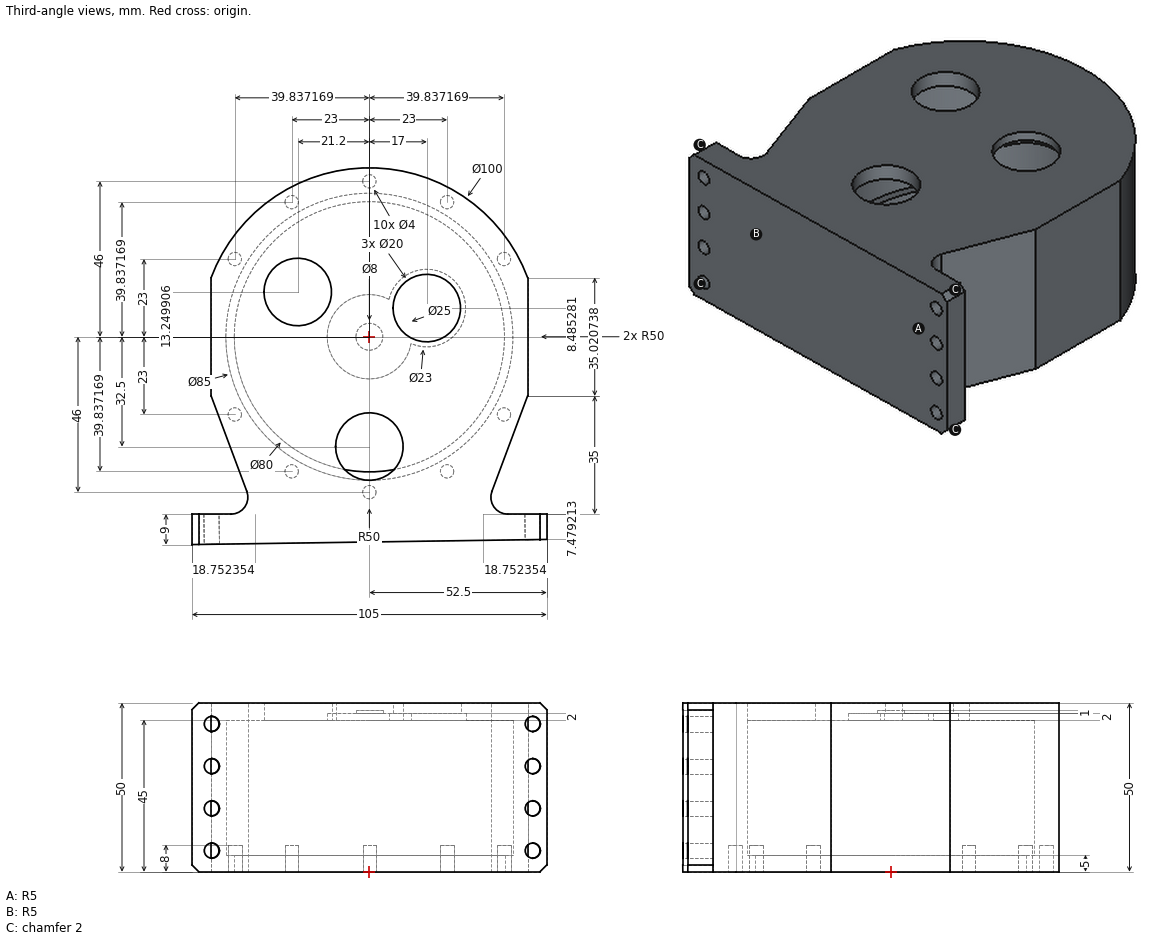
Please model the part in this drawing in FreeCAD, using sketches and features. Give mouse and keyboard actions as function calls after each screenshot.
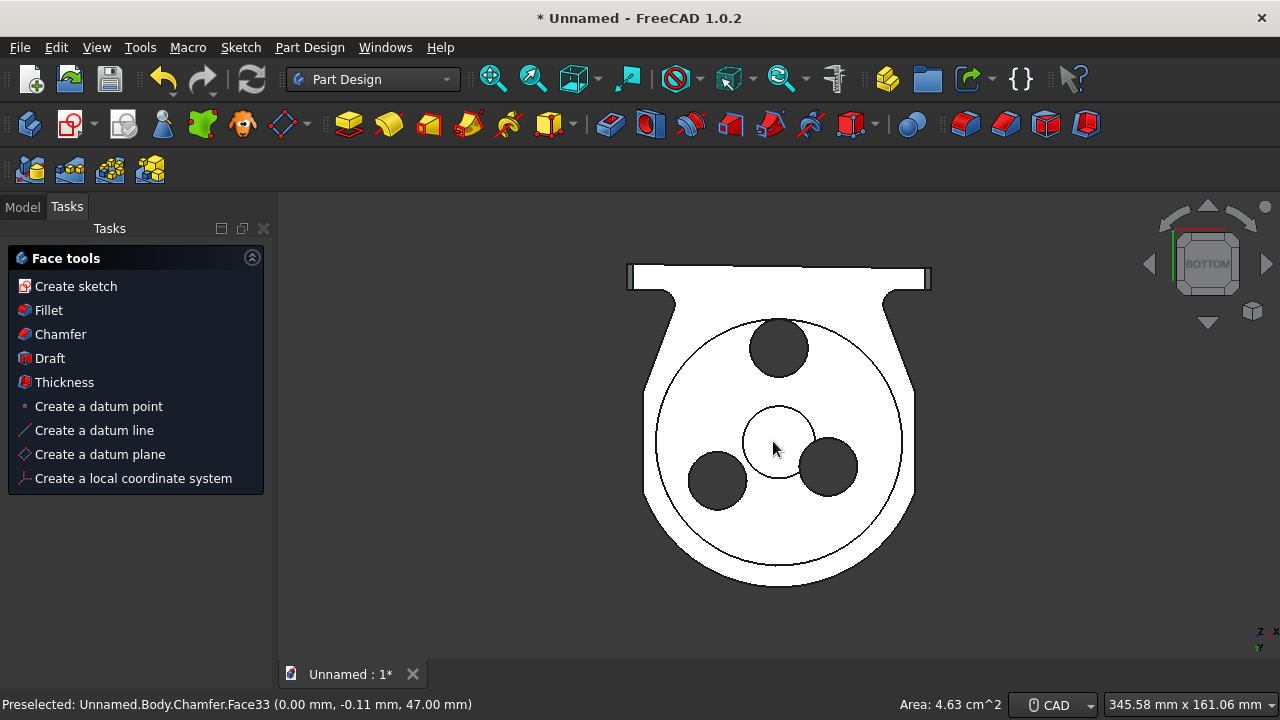
click(70, 124)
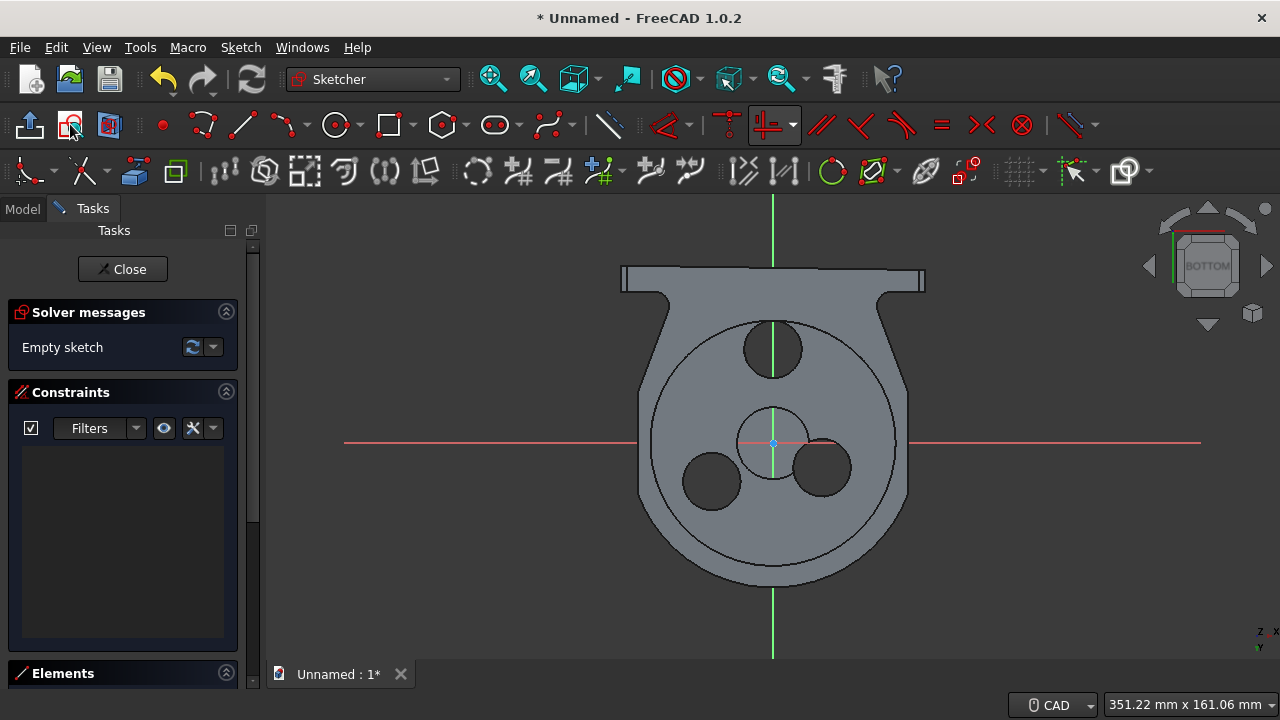
scroll(778, 445, up, 13)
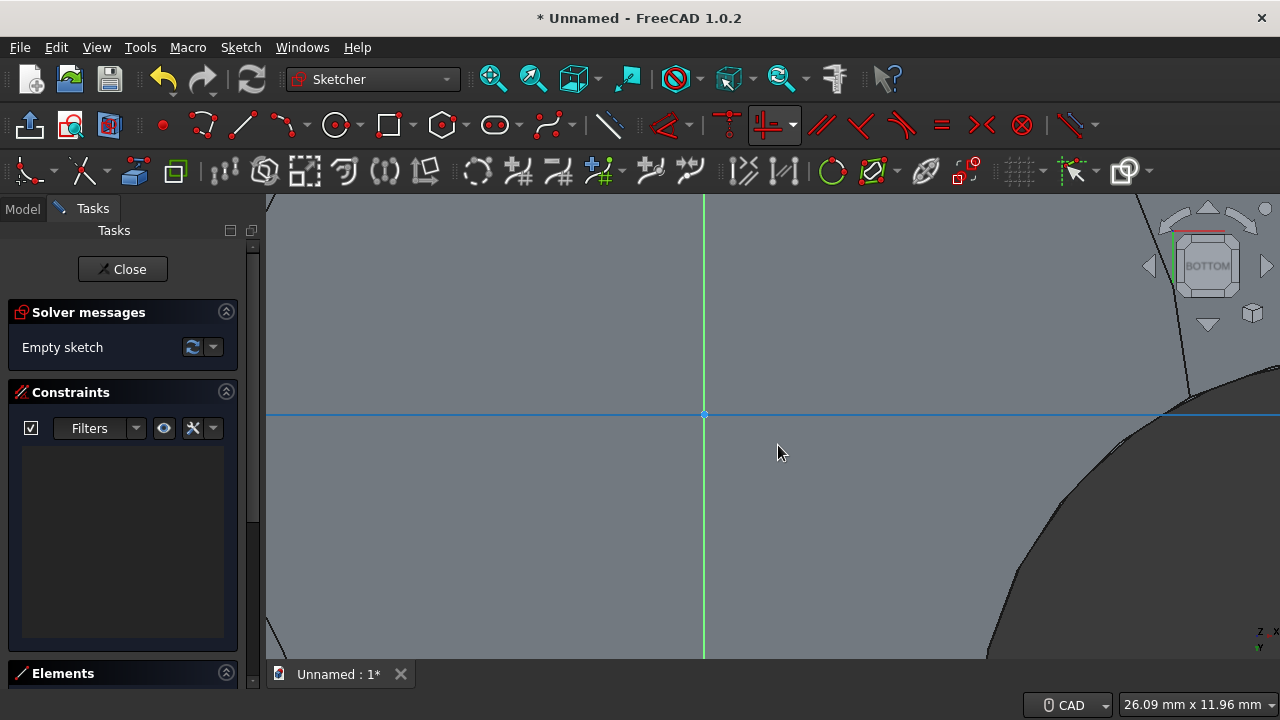
click(336, 126)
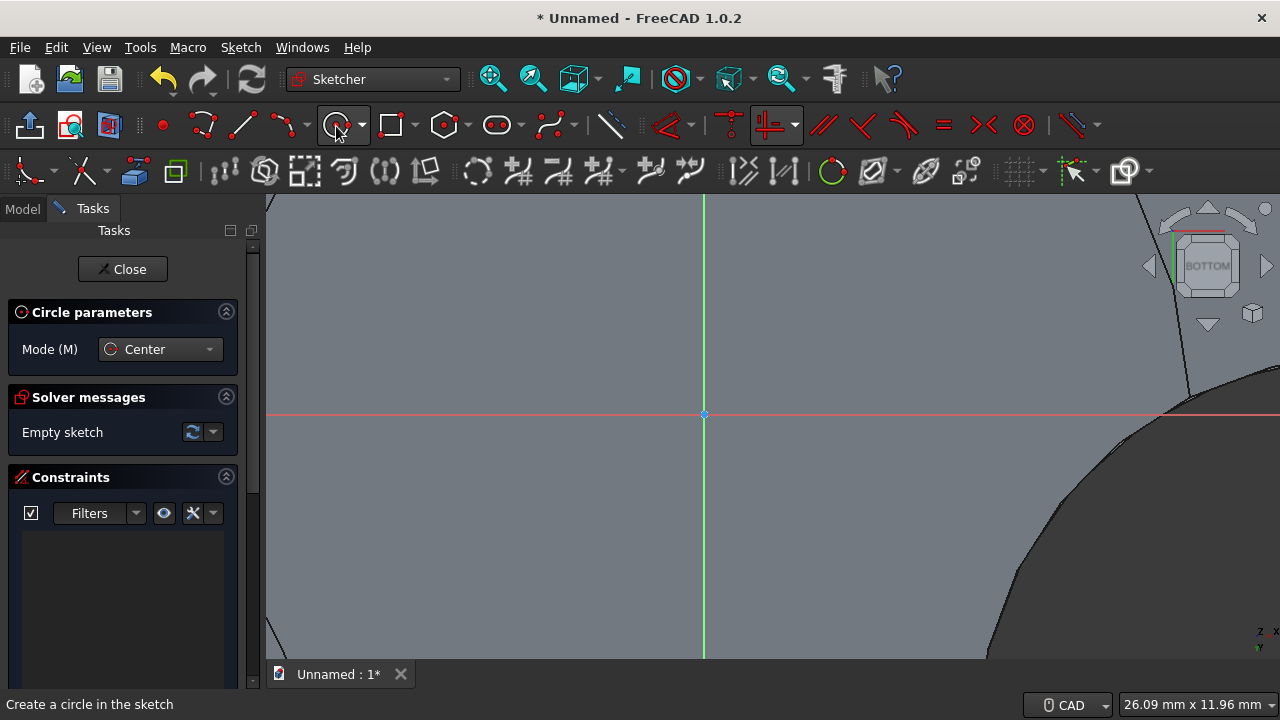
click(704, 415)
click(814, 305)
key(Escape)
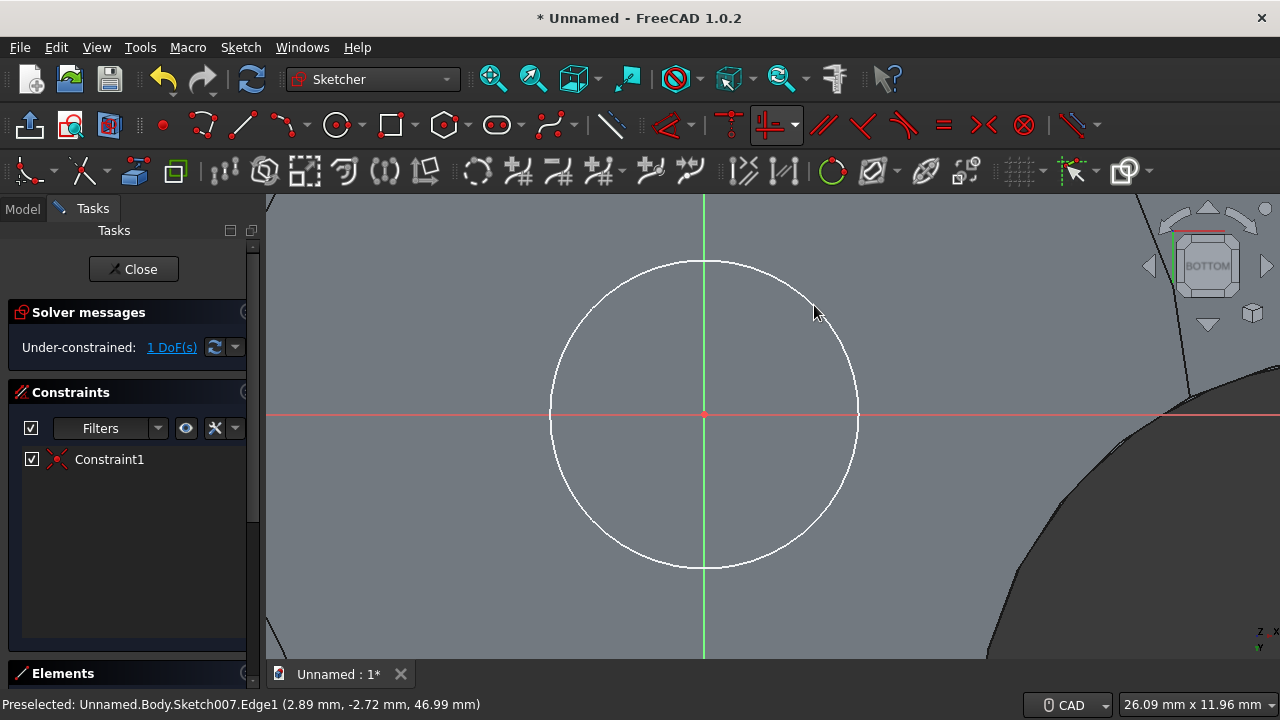
click(666, 126)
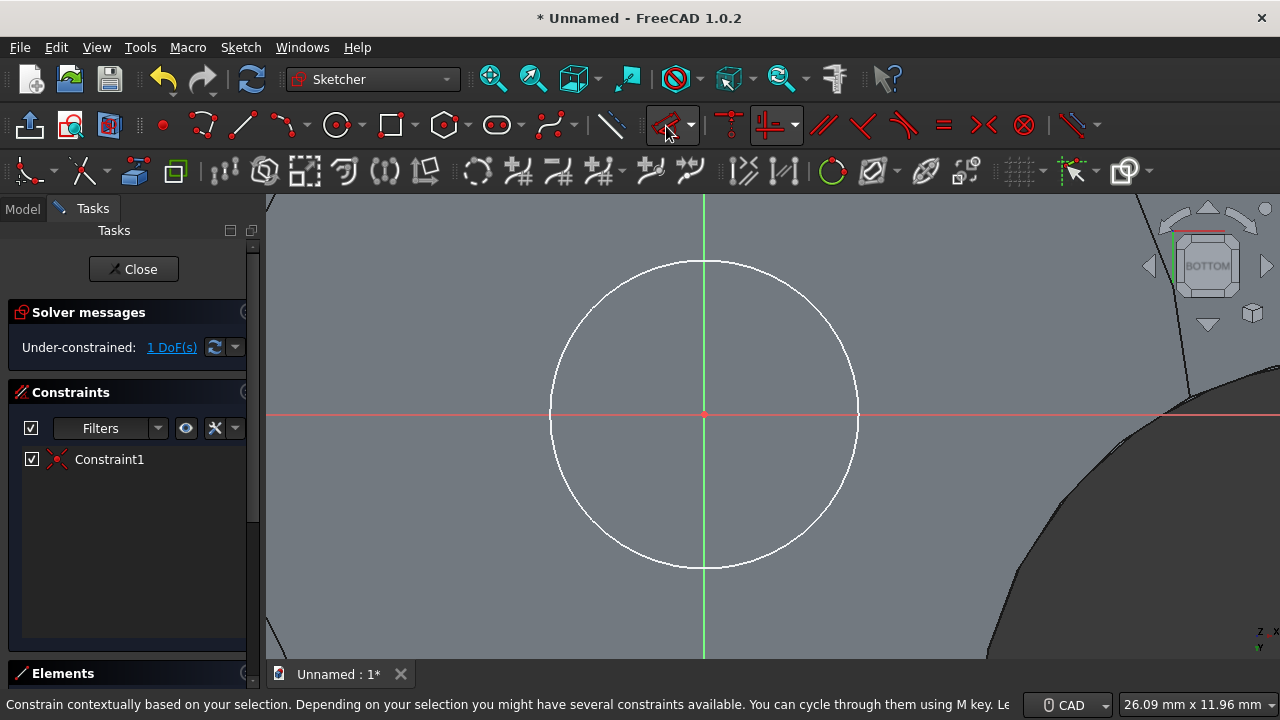
click(813, 305)
click(836, 282)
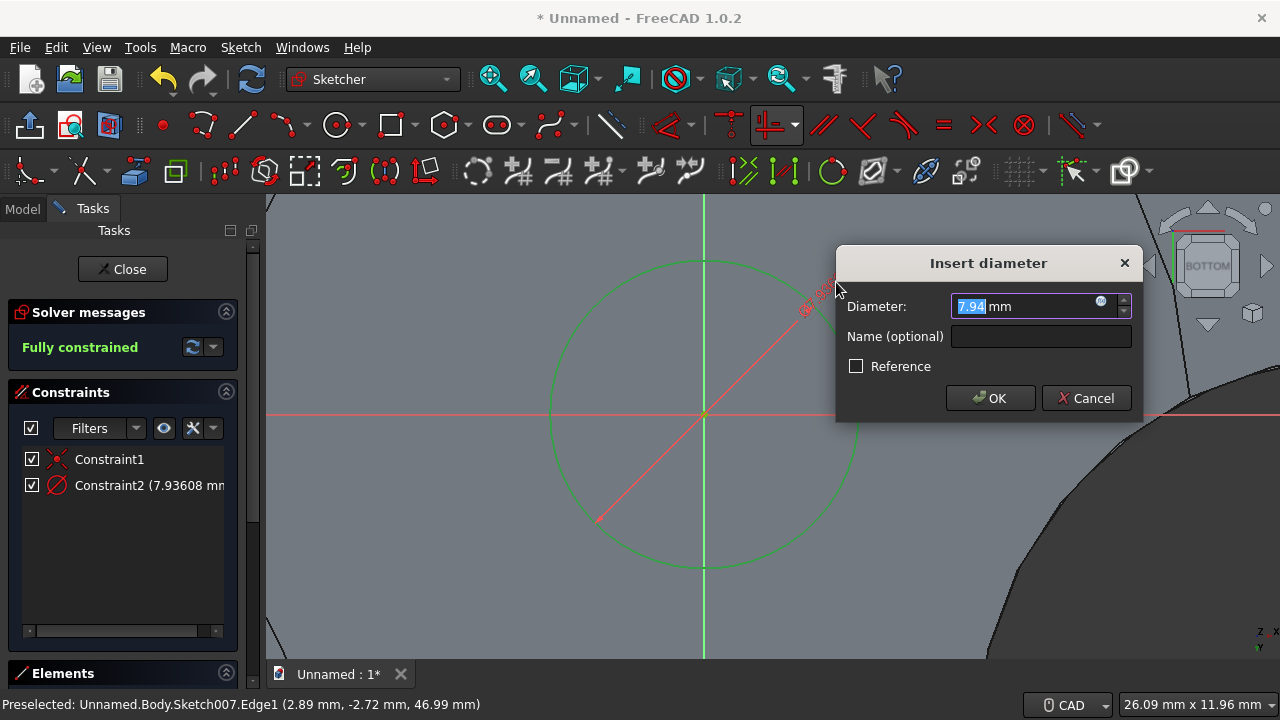
text(8)
key(Return)
key(Escape)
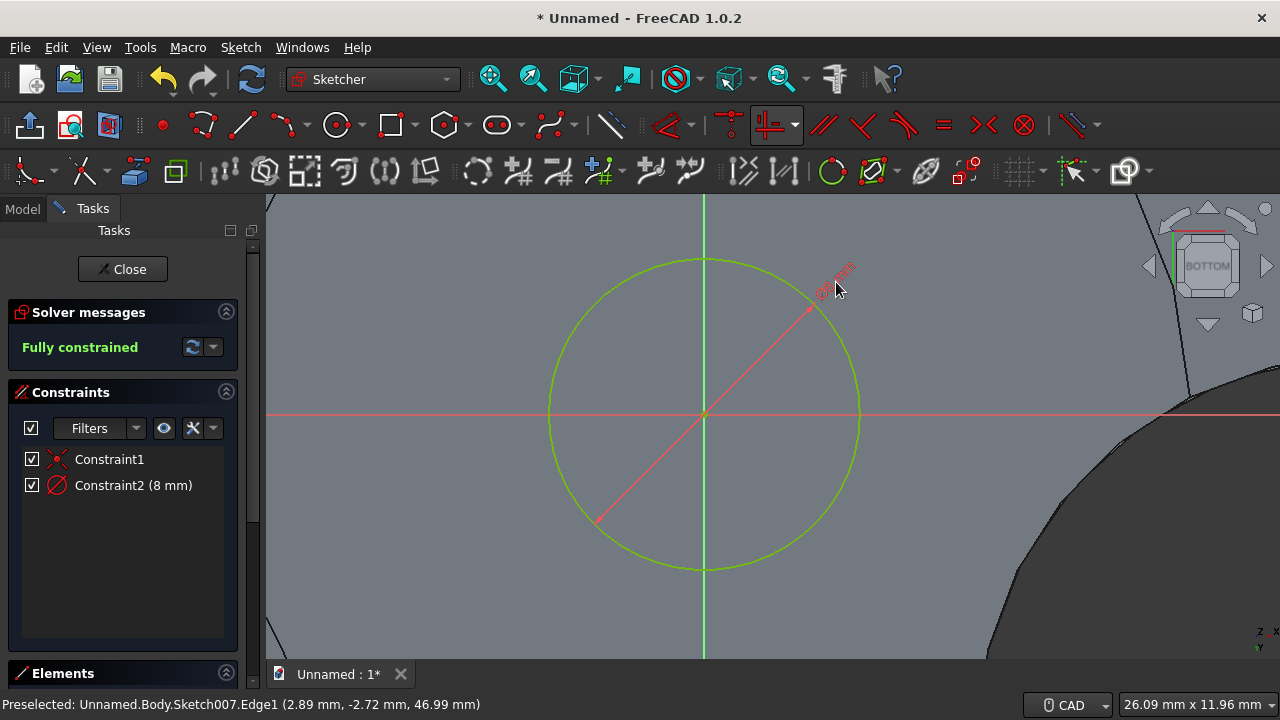
click(123, 269)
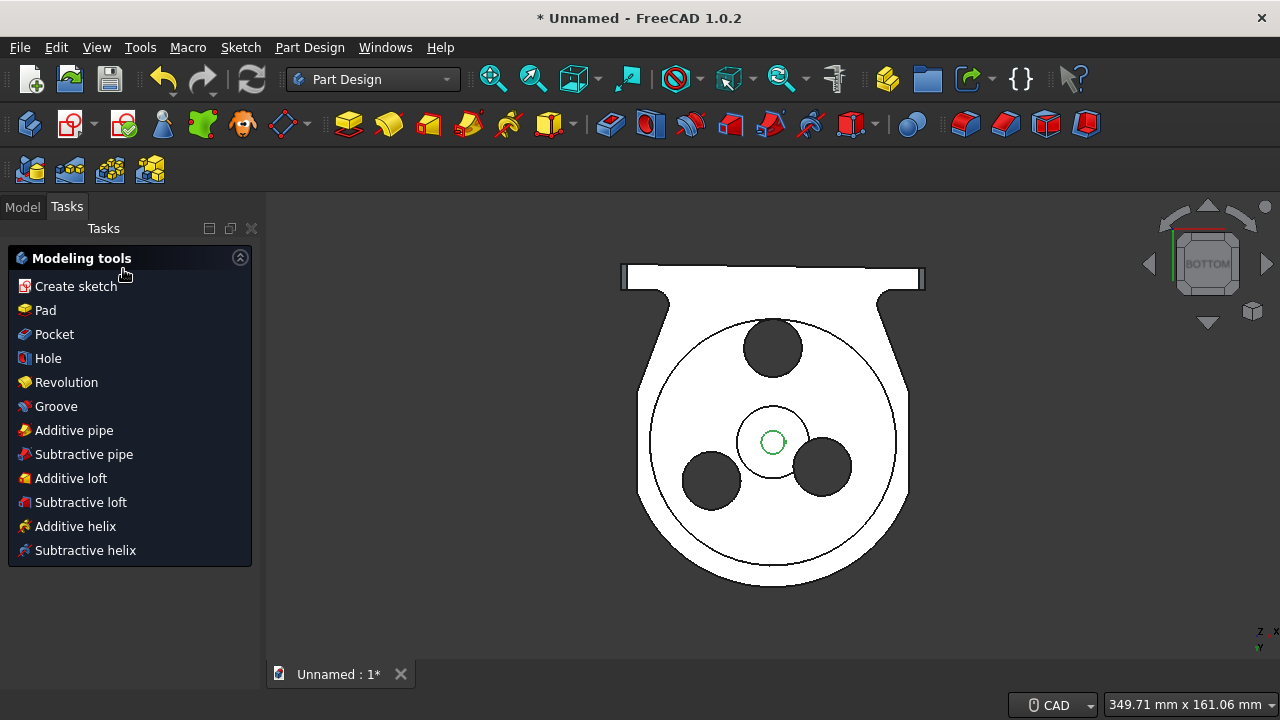
click(612, 124)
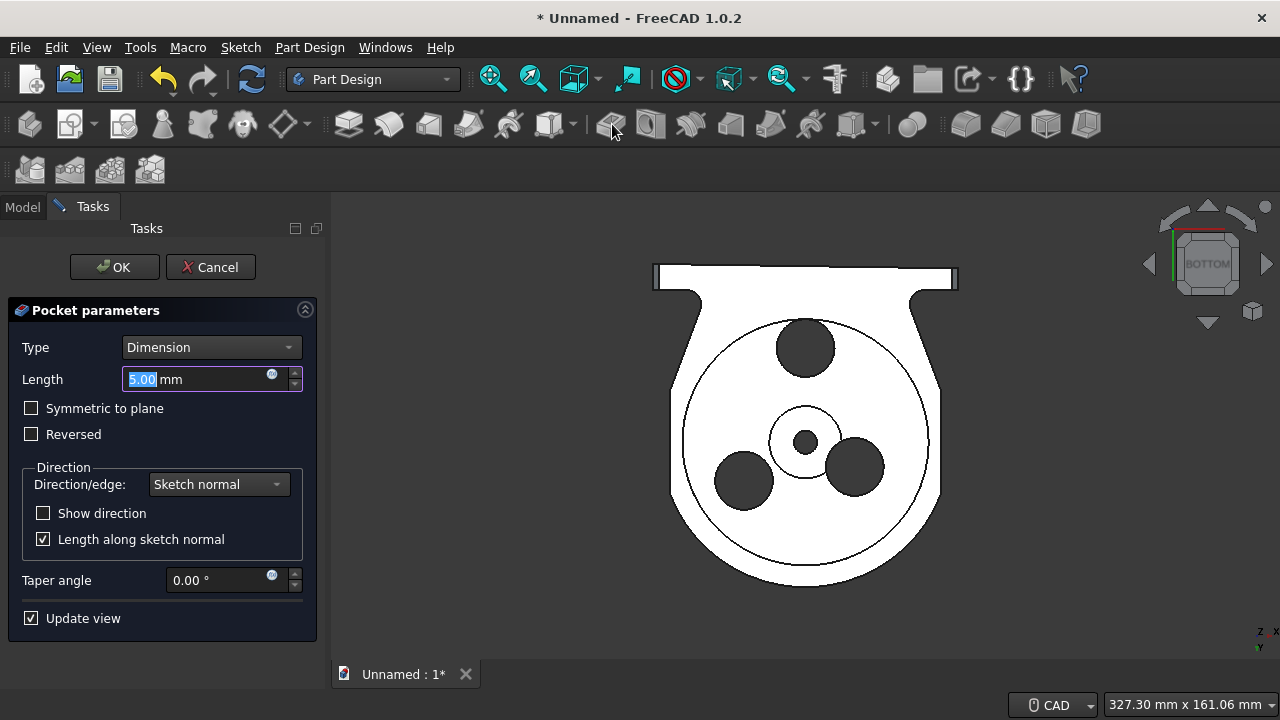
text(1)
key(Tab)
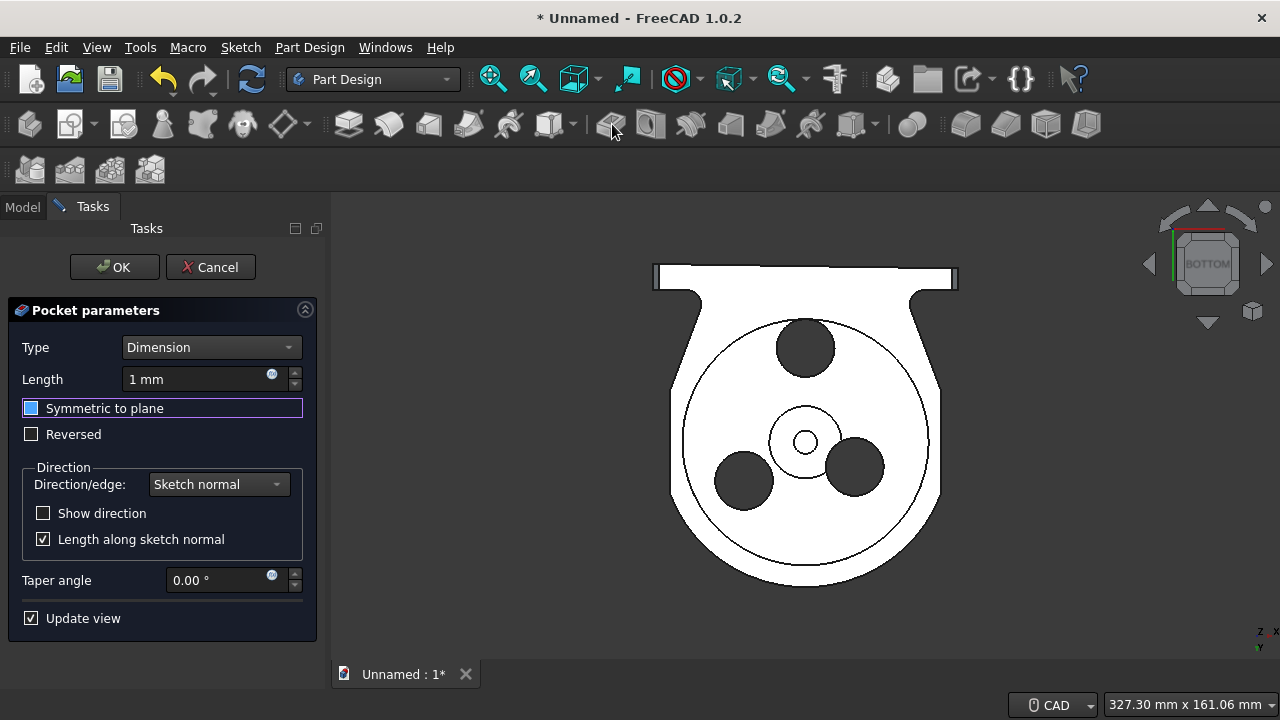
click(115, 267)